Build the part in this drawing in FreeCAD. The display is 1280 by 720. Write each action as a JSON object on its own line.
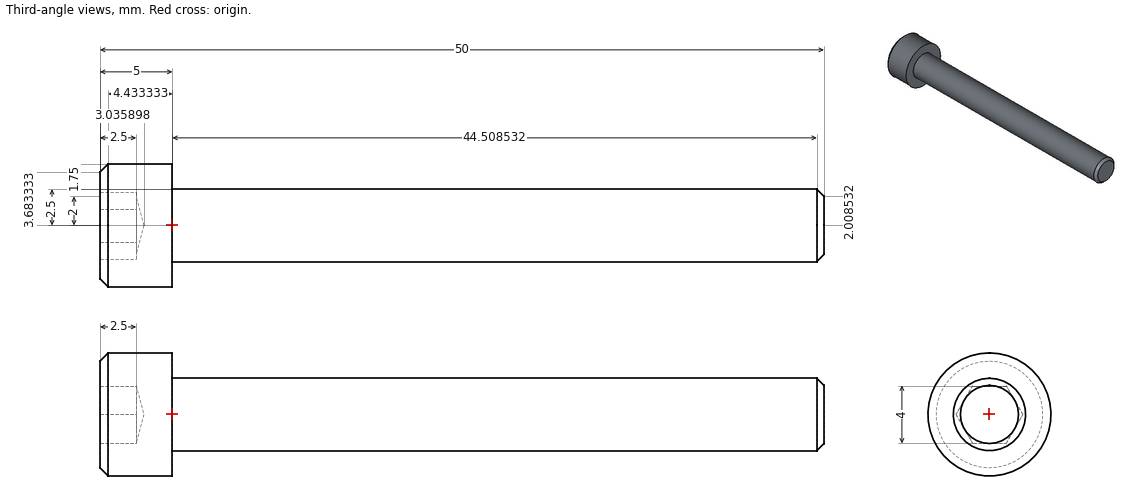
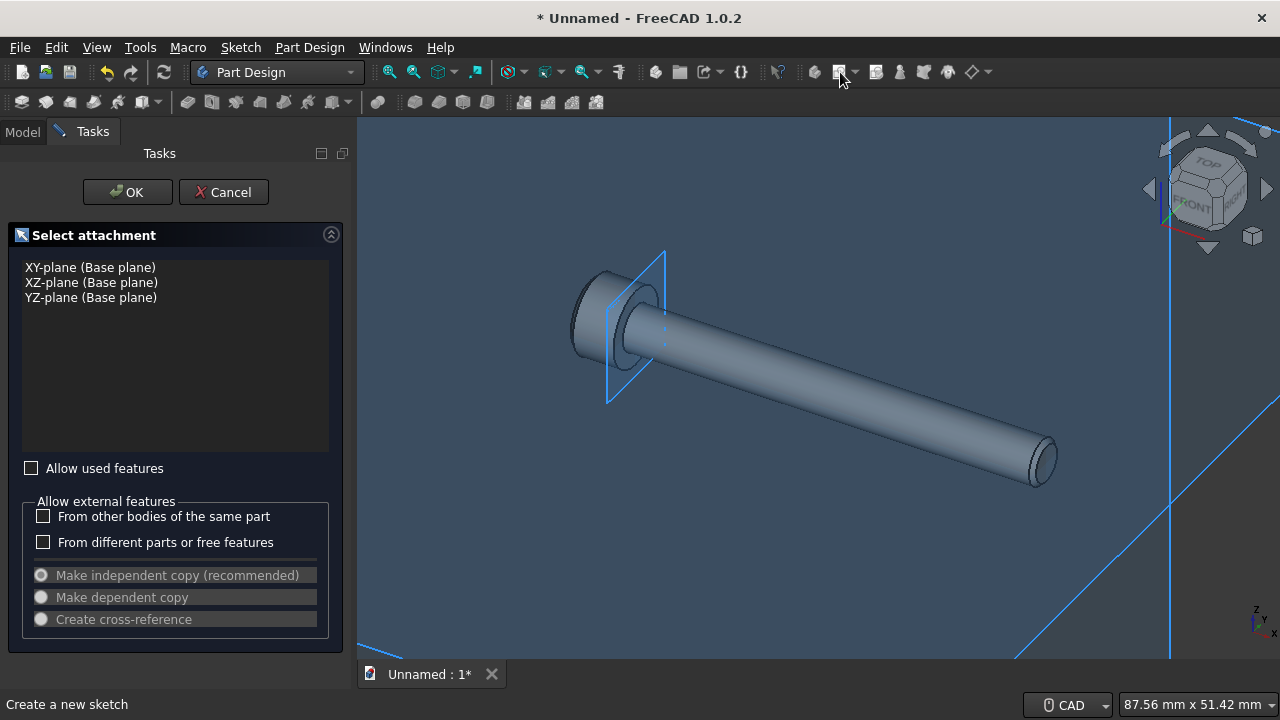
{"action": "left_click", "coordinate": [82, 268]}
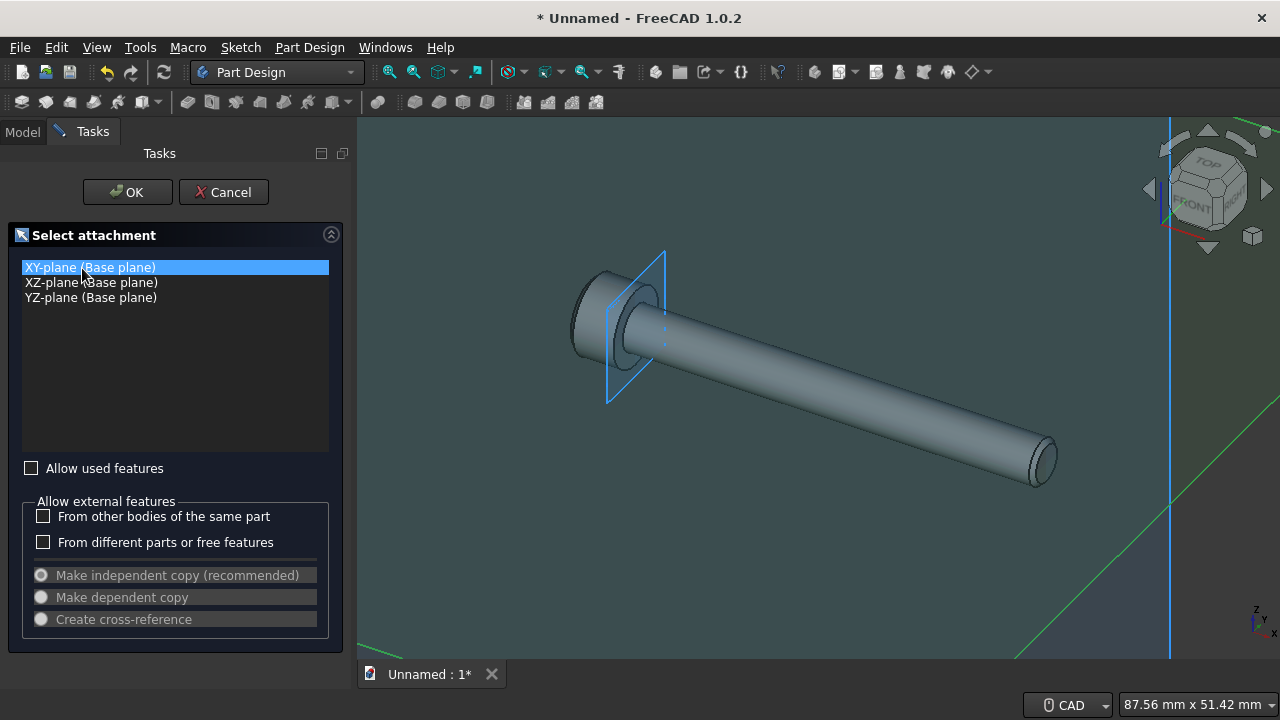
{"action": "left_click", "coordinate": [128, 192]}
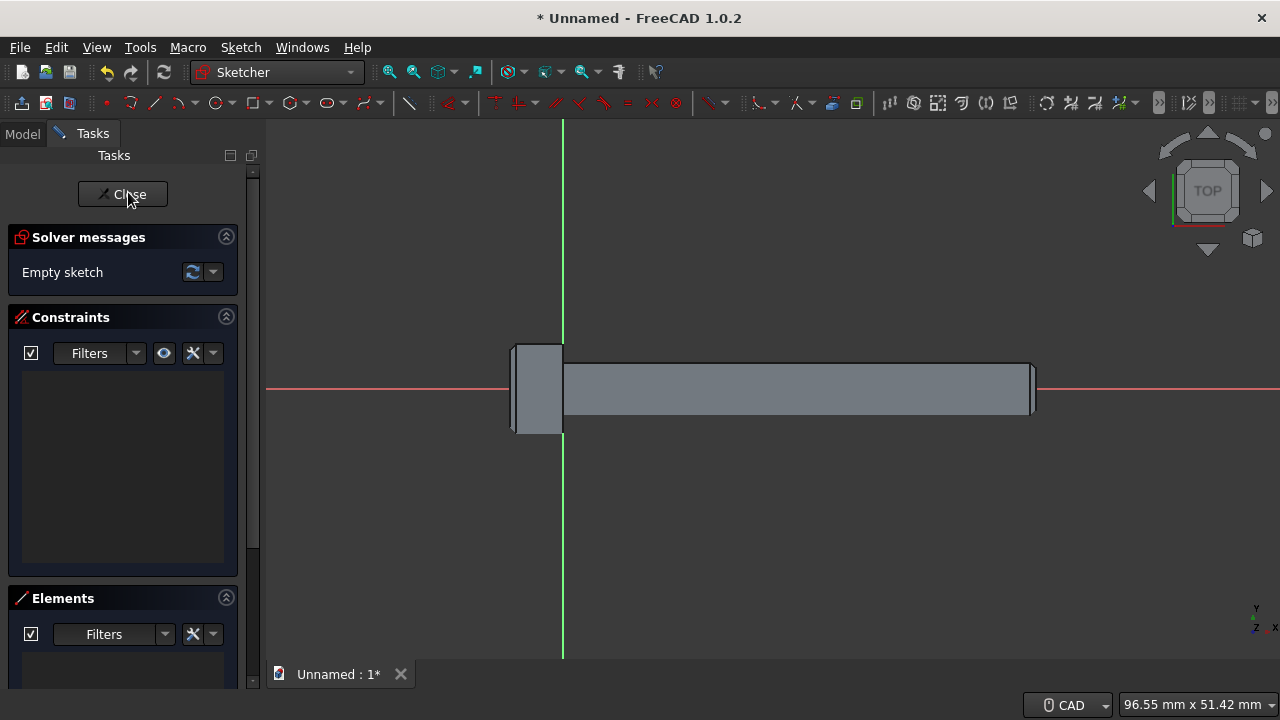
{"action": "key", "text": "q s"}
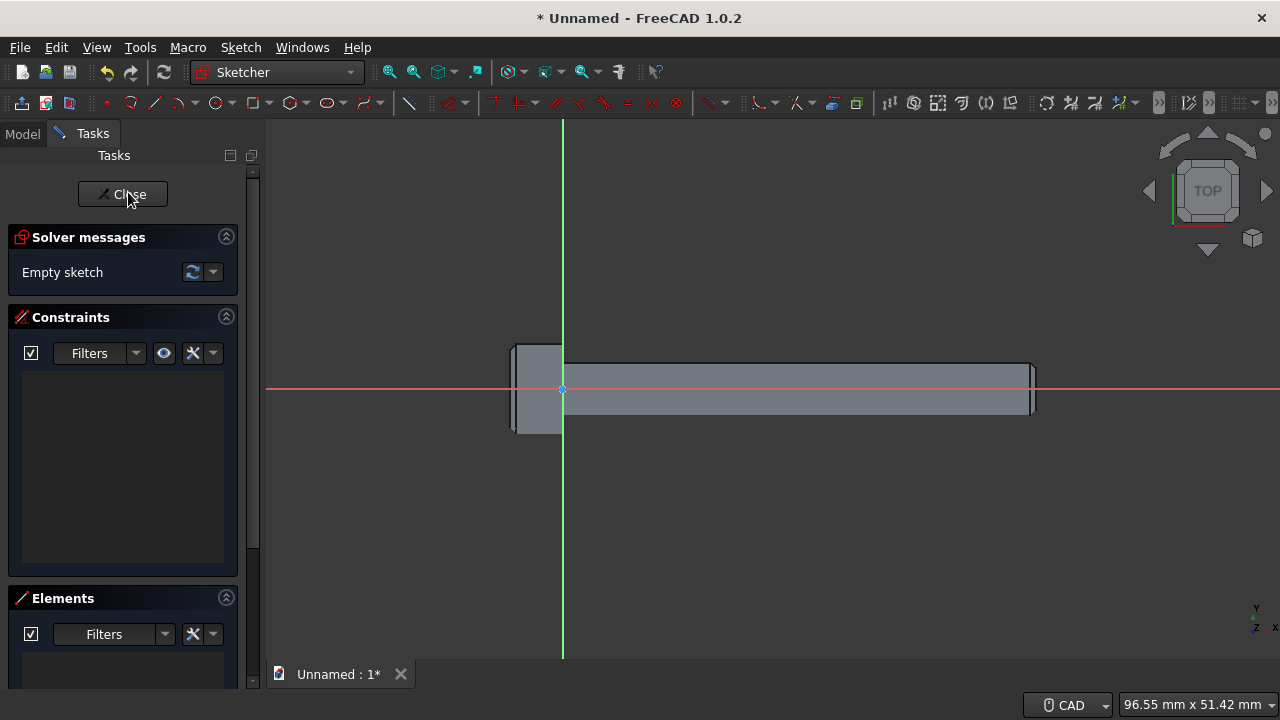
{"action": "scroll", "coordinate": [520, 378], "scroll_direction": "up", "scroll_amount": 12}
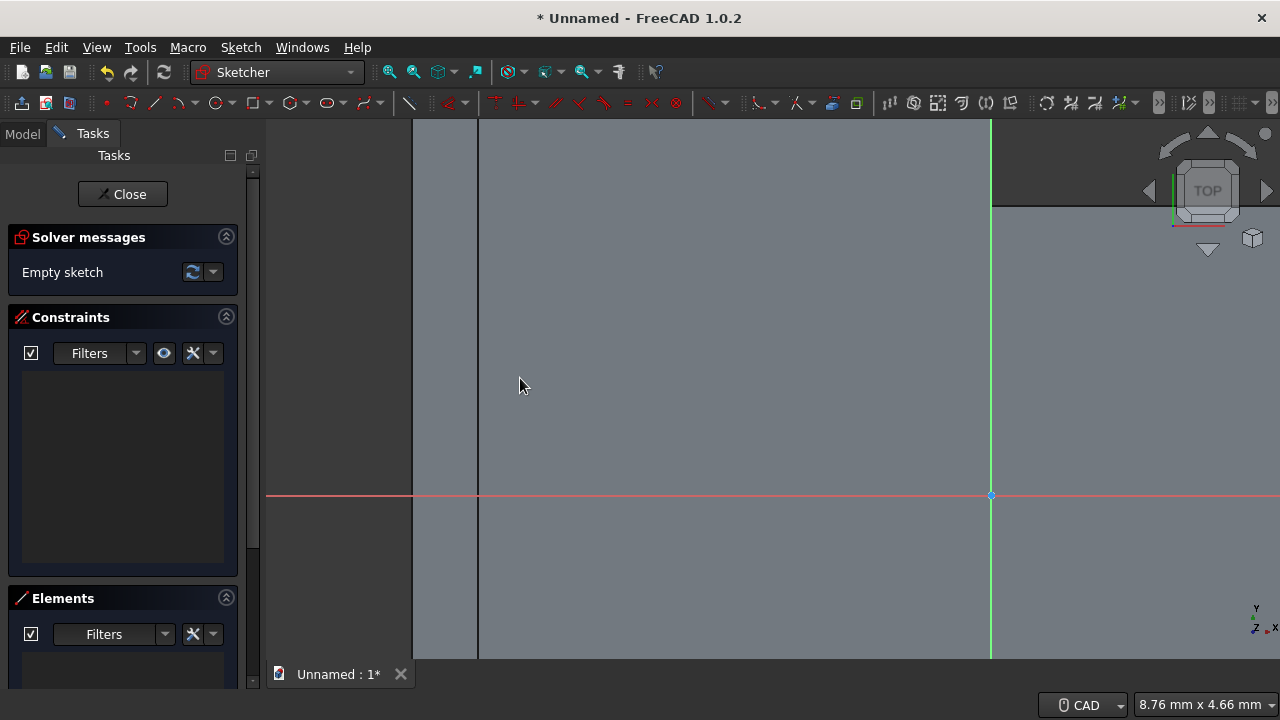
{"action": "left_click", "coordinate": [132, 104]}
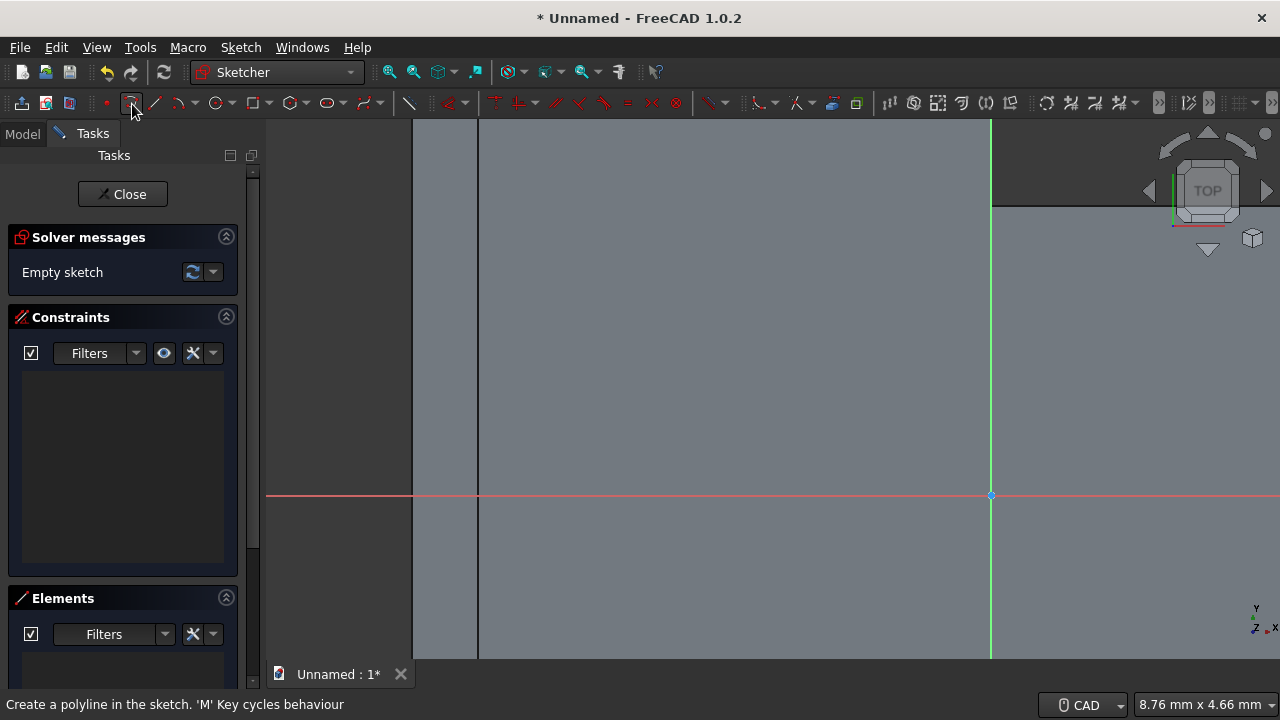
{"action": "left_click", "coordinate": [764, 496]}
{"action": "left_click", "coordinate": [702, 264]}
{"action": "left_click", "coordinate": [412, 264]}
{"action": "left_click", "coordinate": [412, 487]}
{"action": "left_click", "coordinate": [764, 496]}
{"action": "key", "text": "Escape"}
{"action": "key", "text": "Escape"}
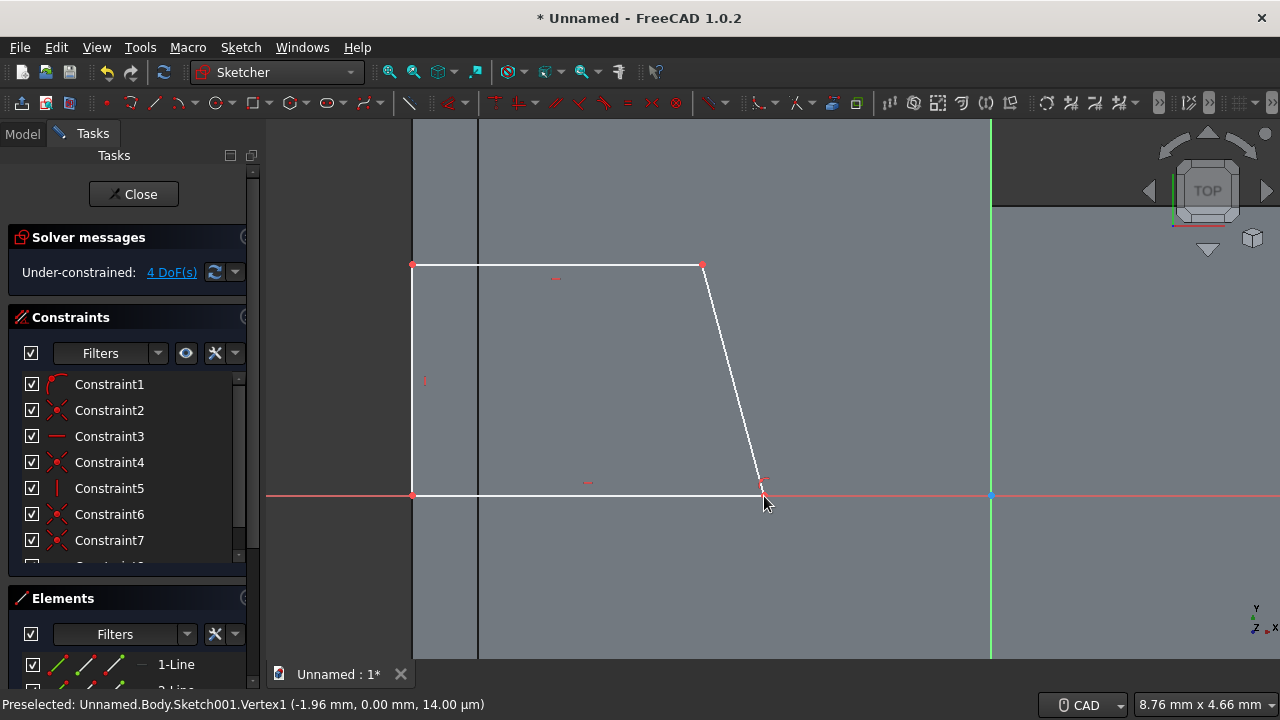
{"action": "left_click", "coordinate": [448, 104]}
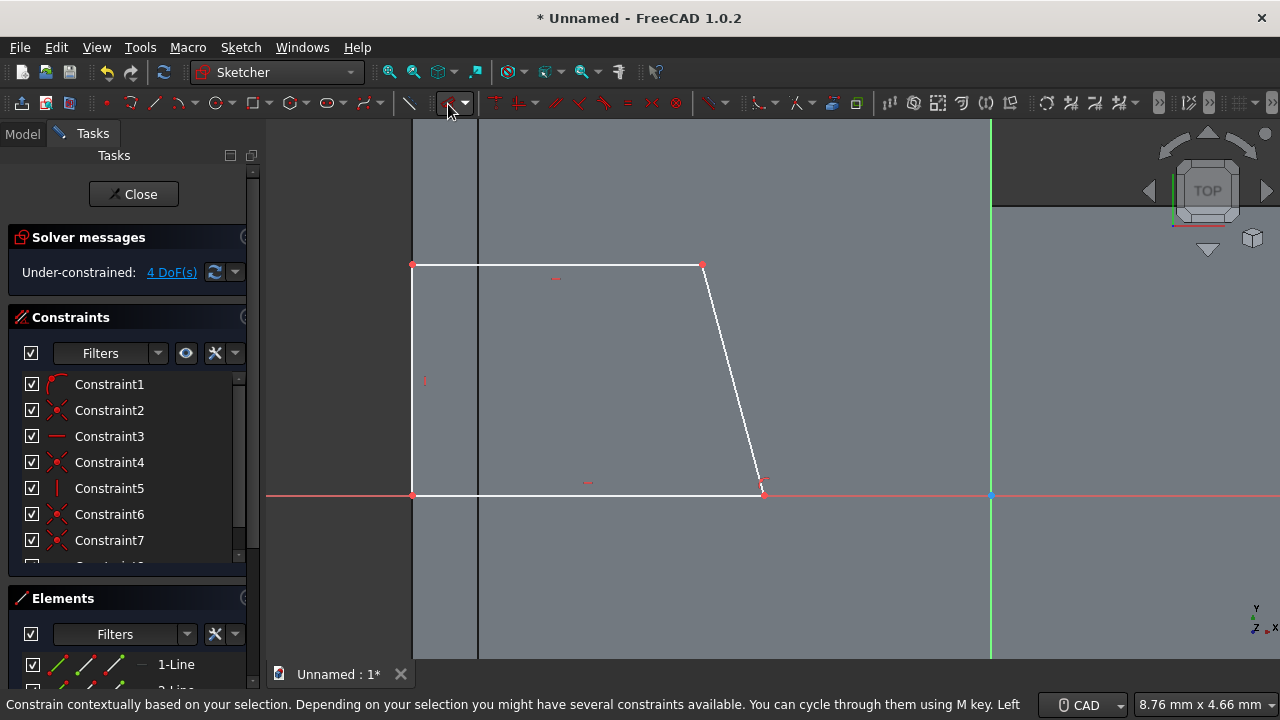
{"action": "left_click", "coordinate": [412, 334]}
{"action": "left_click", "coordinate": [378, 380]}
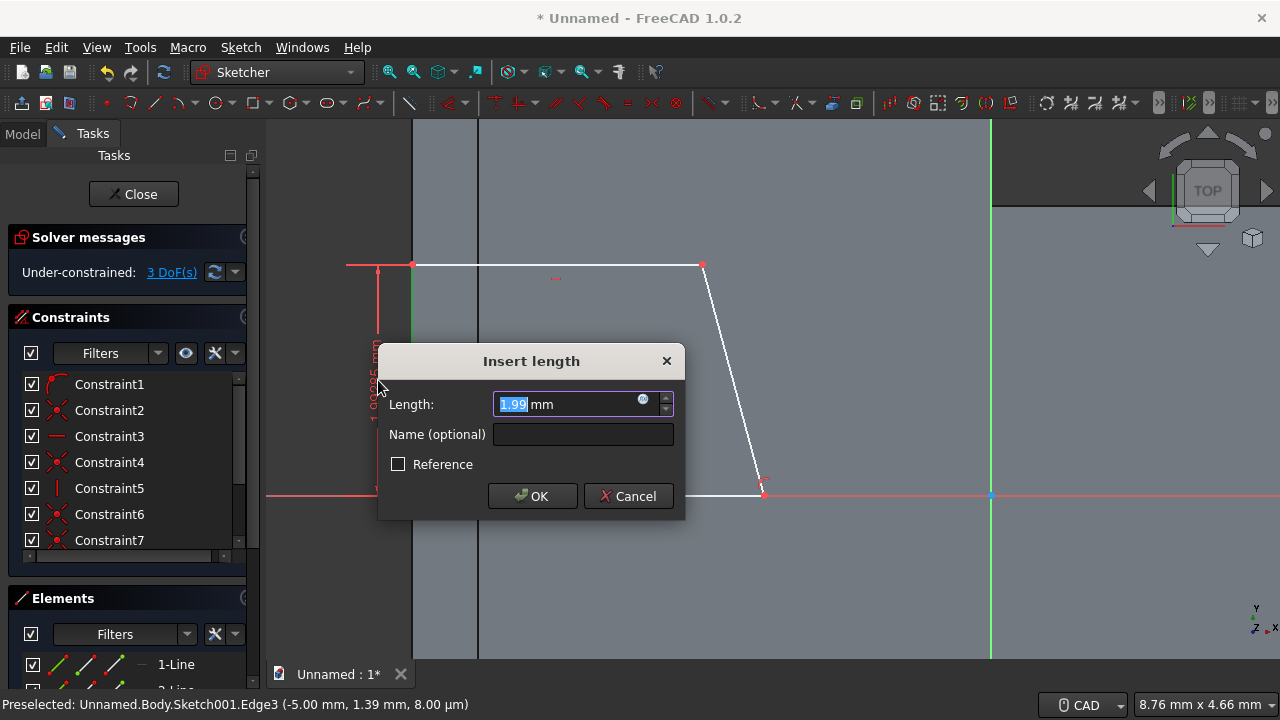
{"action": "type", "text": "2"}
{"action": "key", "text": "Return"}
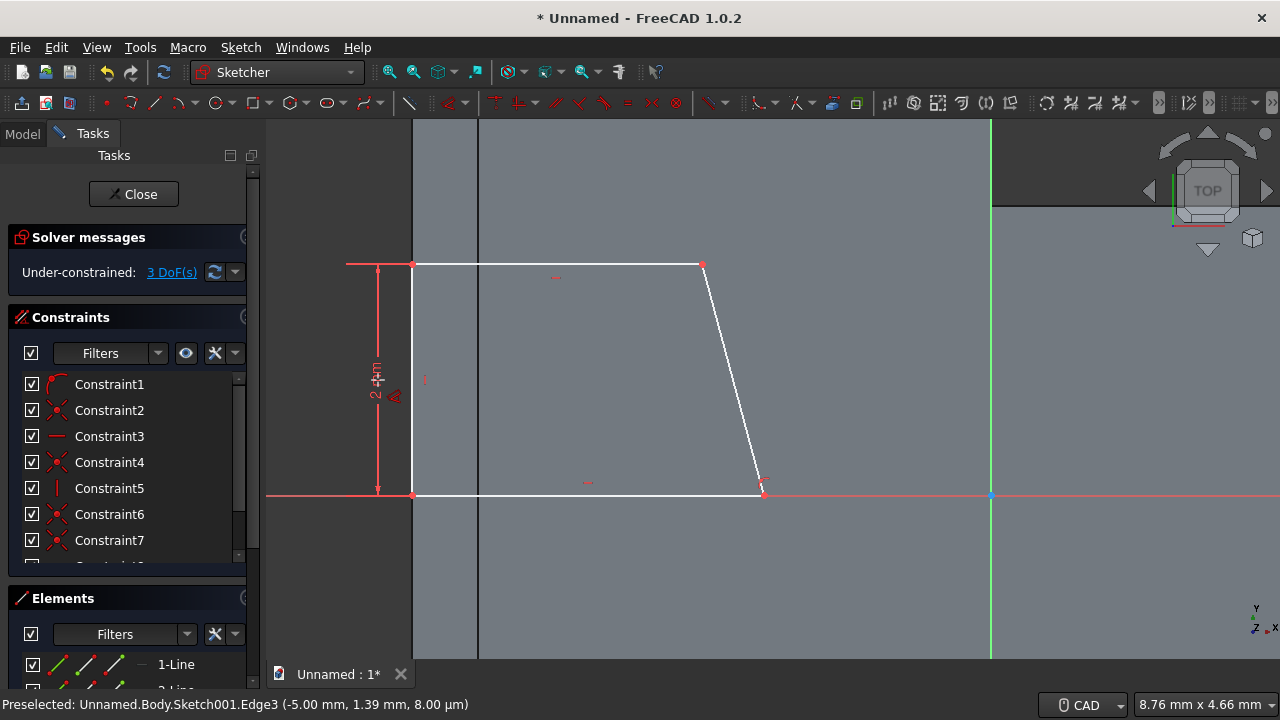
{"action": "left_click", "coordinate": [412, 264]}
{"action": "left_click", "coordinate": [702, 530]}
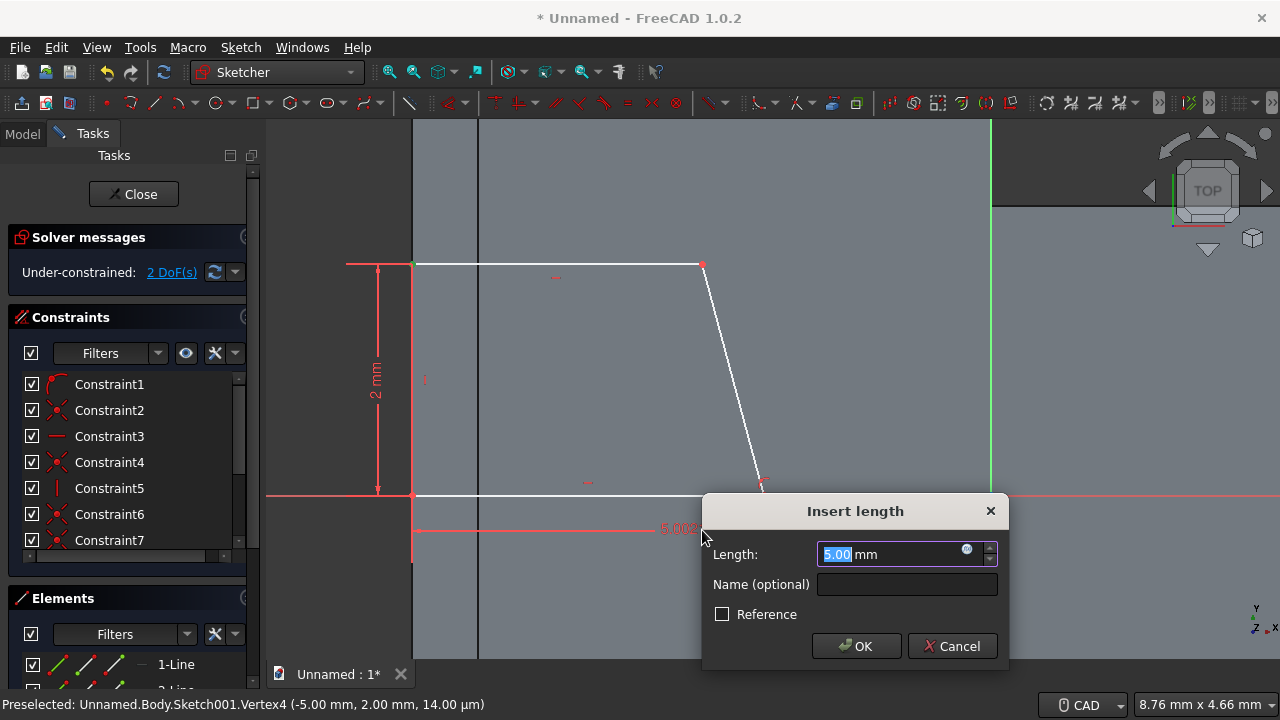
{"action": "type", "text": "5"}
{"action": "key", "text": "Return"}